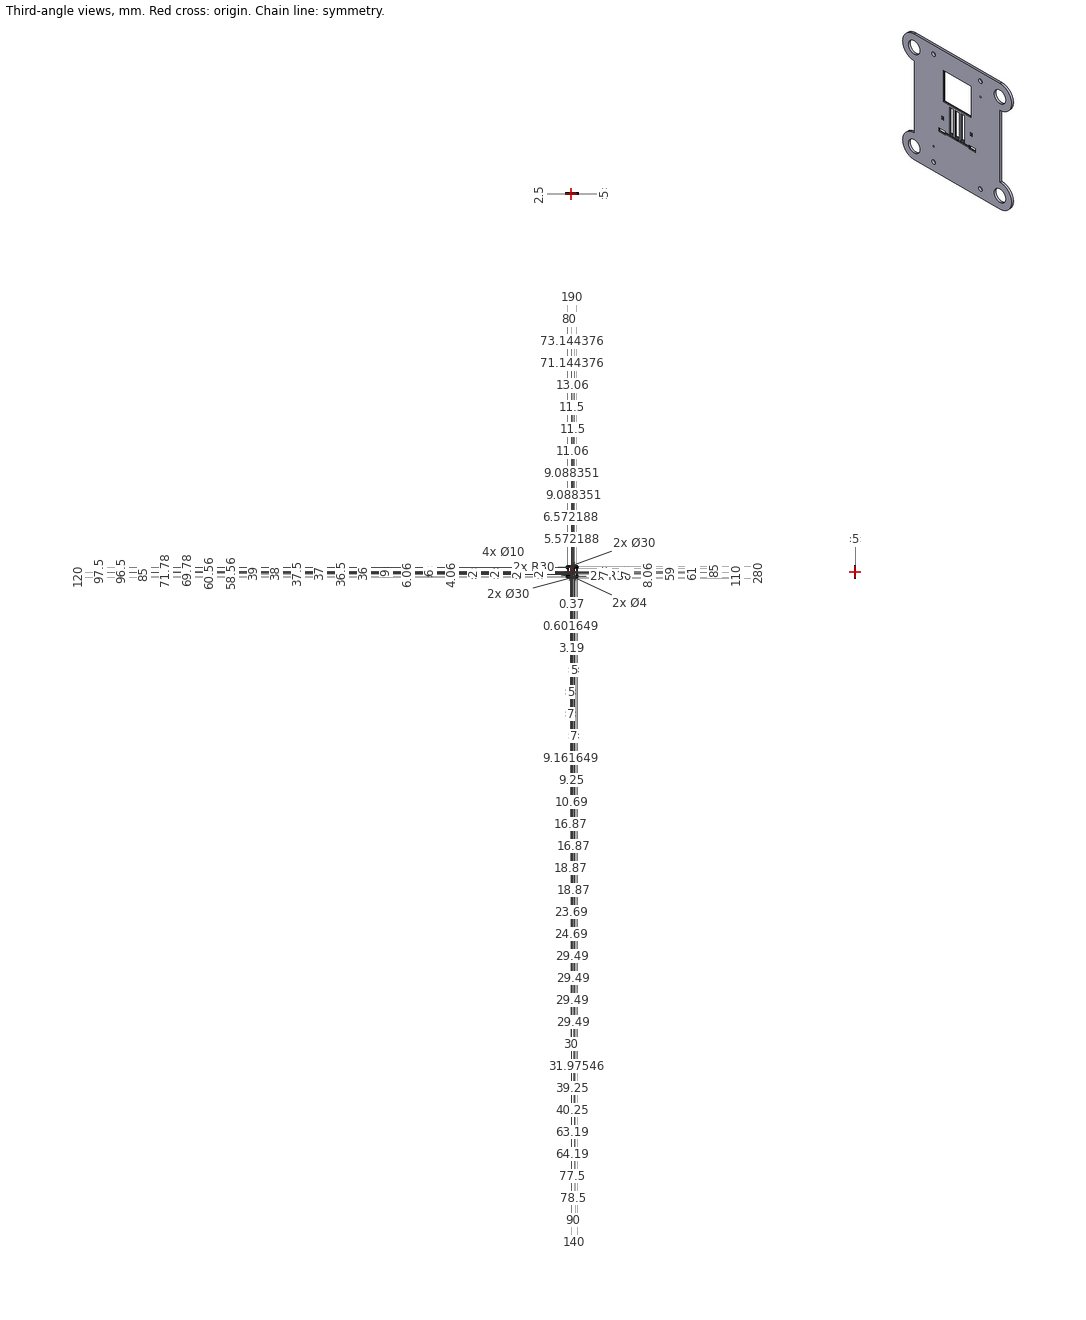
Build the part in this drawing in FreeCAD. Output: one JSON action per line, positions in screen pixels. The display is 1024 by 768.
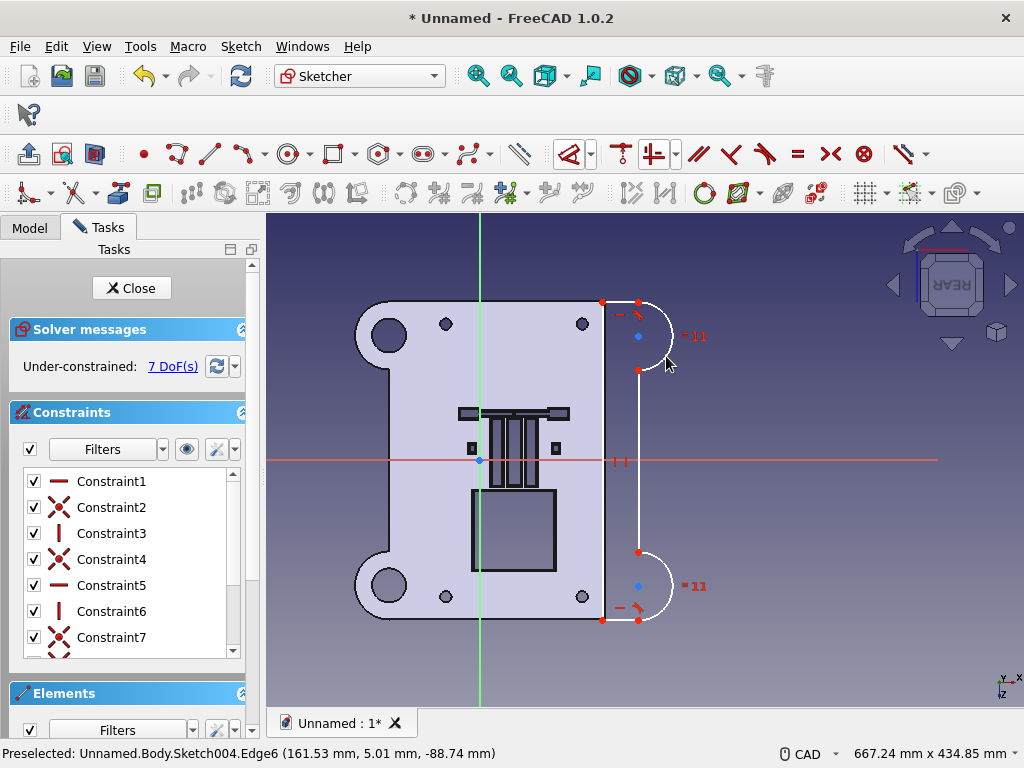
{"action": "left_click", "coordinate": [639, 586]}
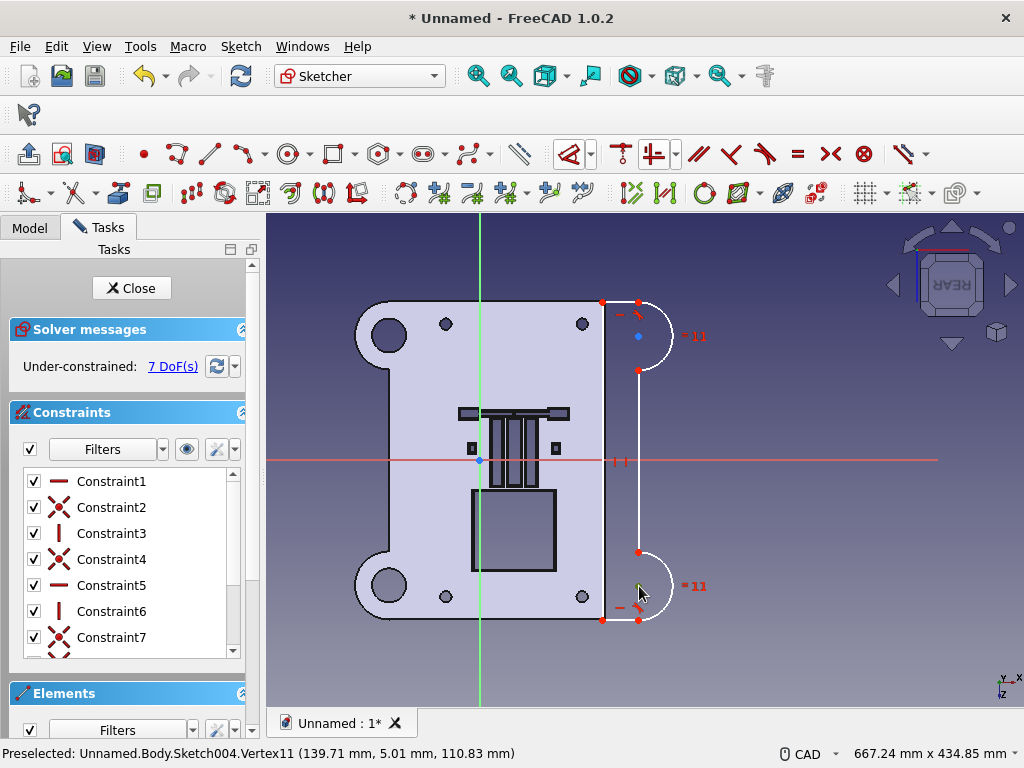
{"action": "left_click", "coordinate": [639, 336]}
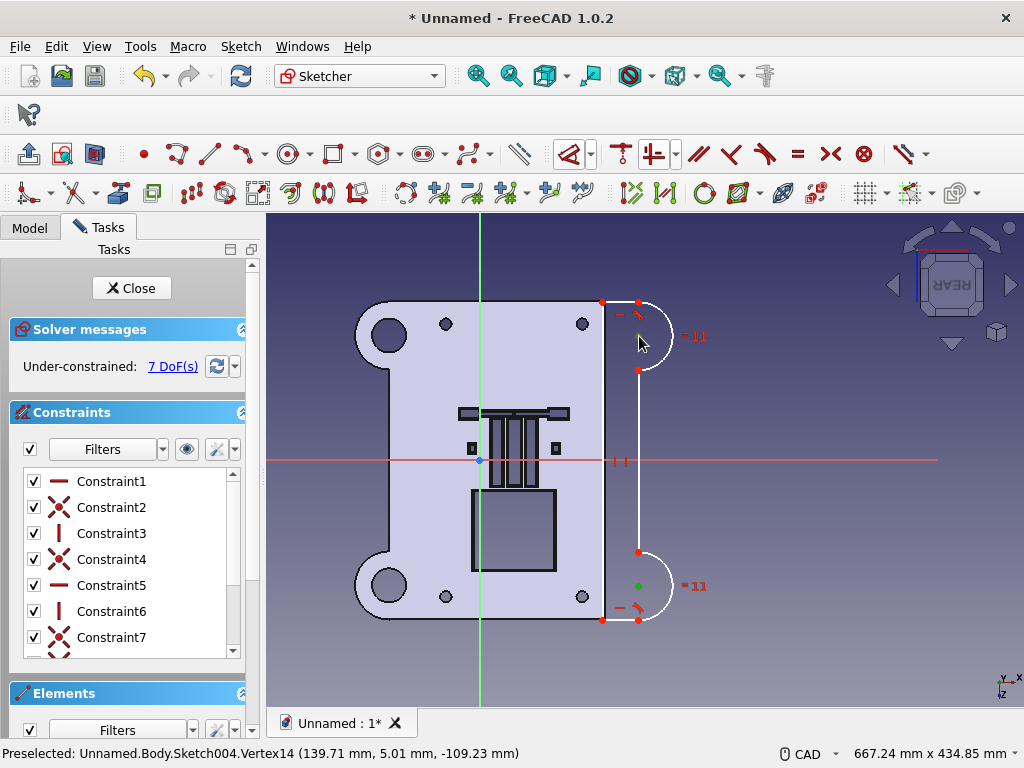
{"action": "left_click", "coordinate": [334, 460]}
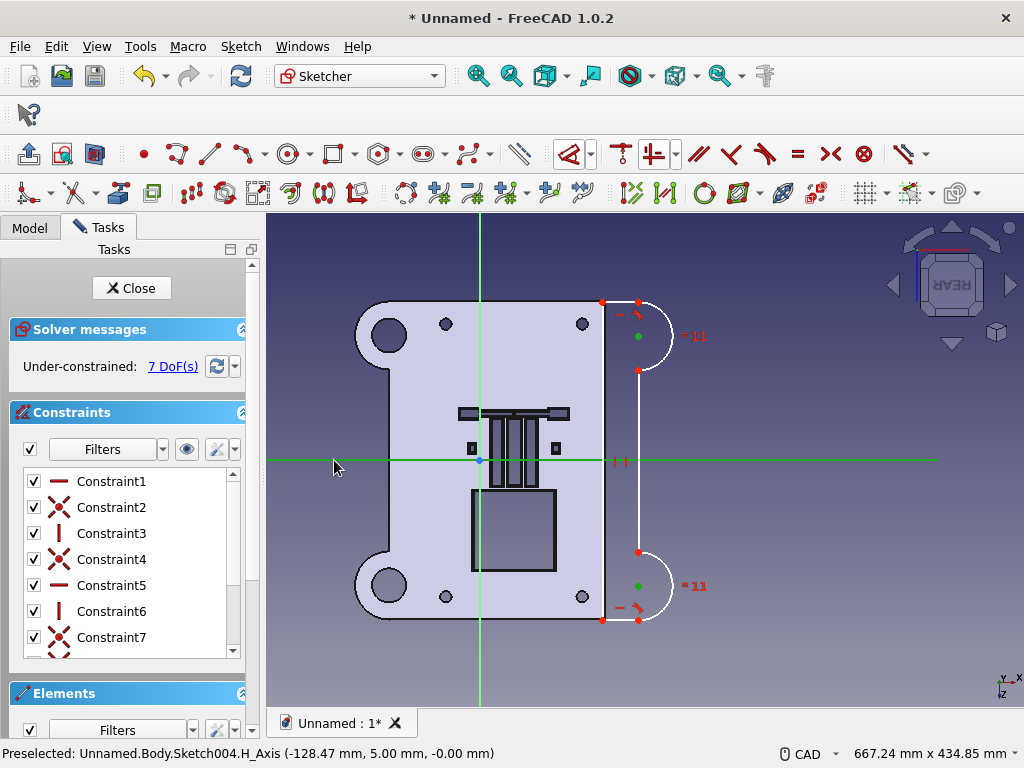
{"action": "left_click", "coordinate": [831, 154]}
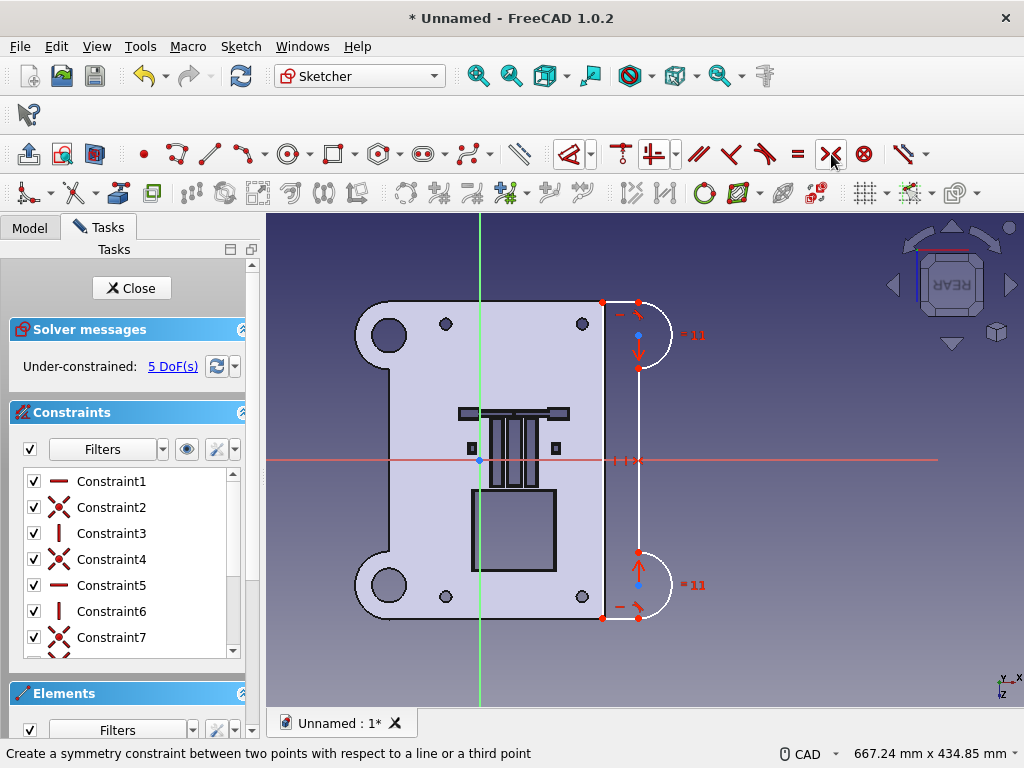
{"action": "left_click", "coordinate": [665, 605]}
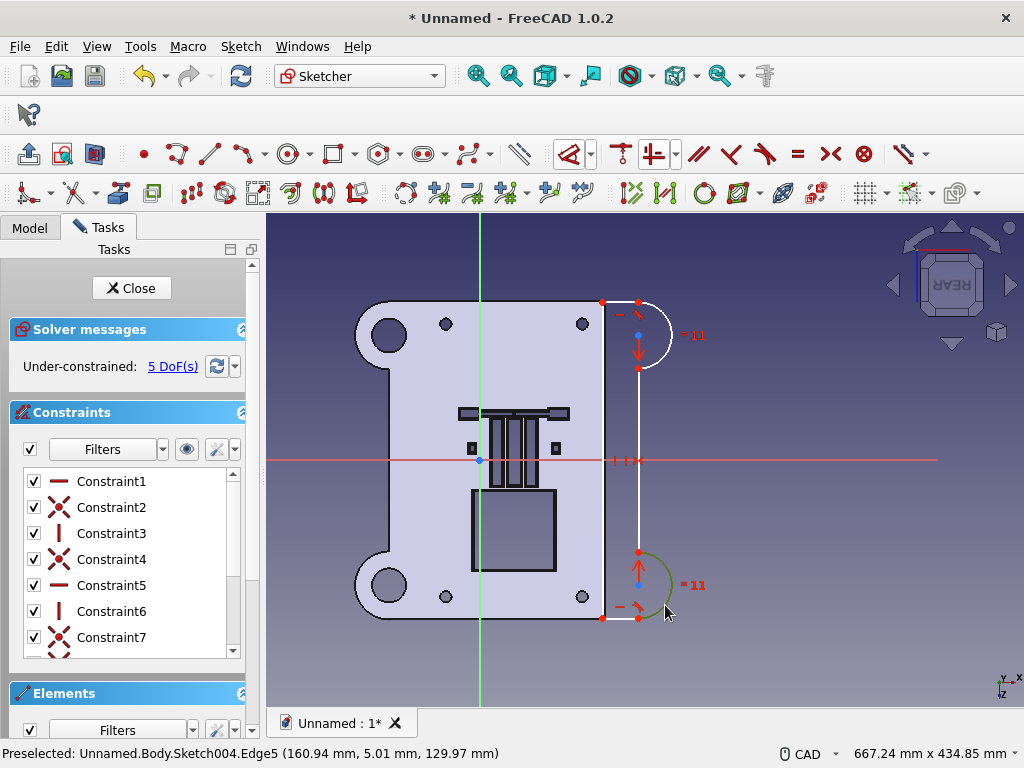
{"action": "left_click", "coordinate": [590, 154]}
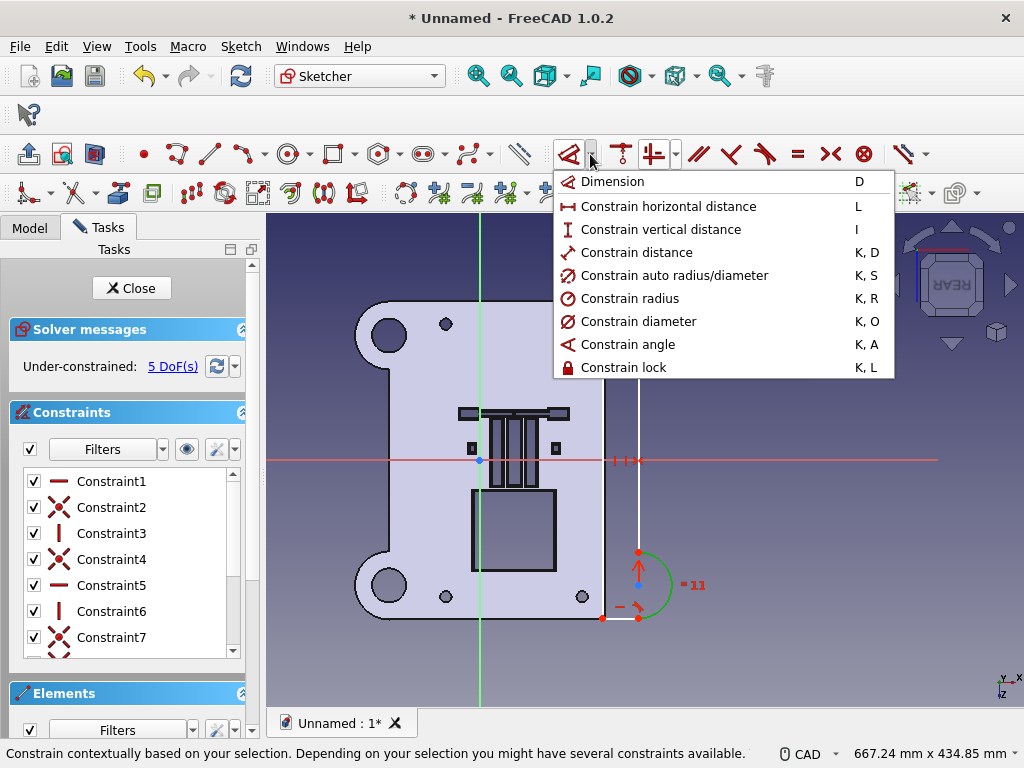
{"action": "left_click", "coordinate": [724, 298]}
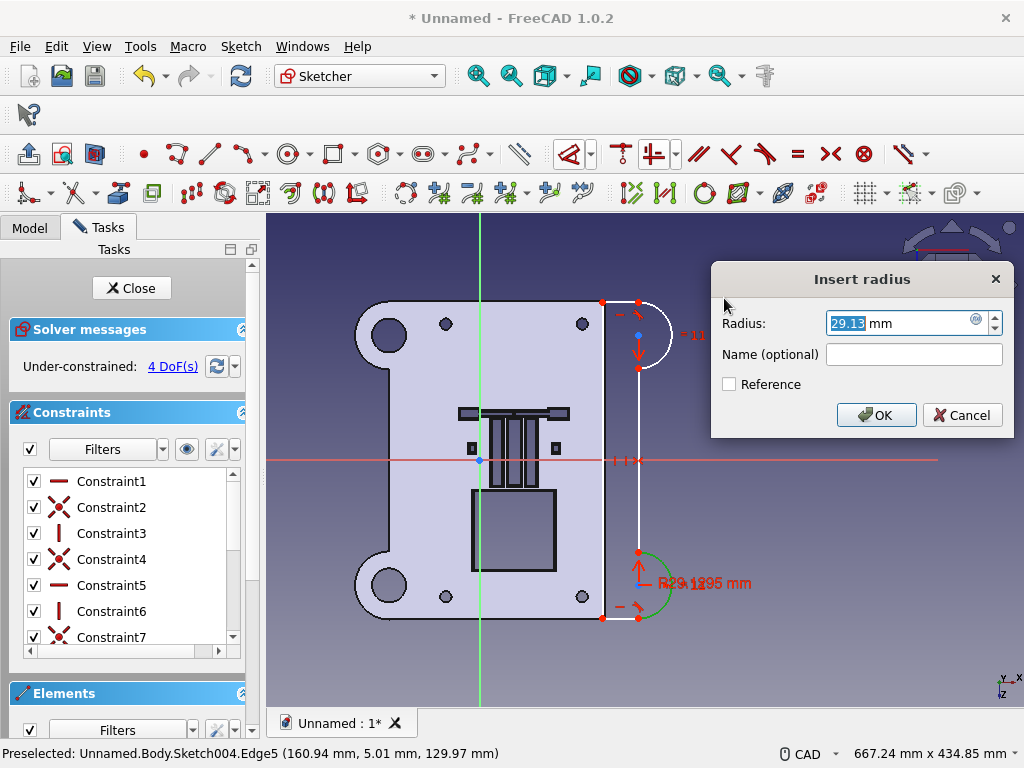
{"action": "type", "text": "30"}
{"action": "key", "text": "Return"}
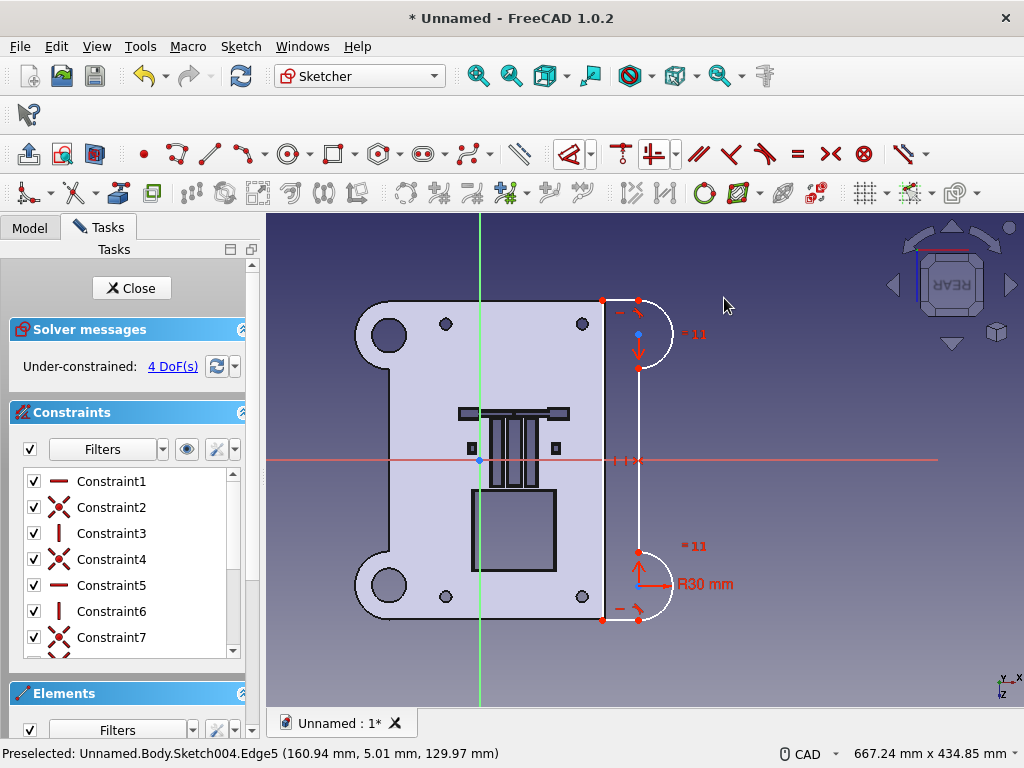
{"action": "left_click", "coordinate": [603, 396]}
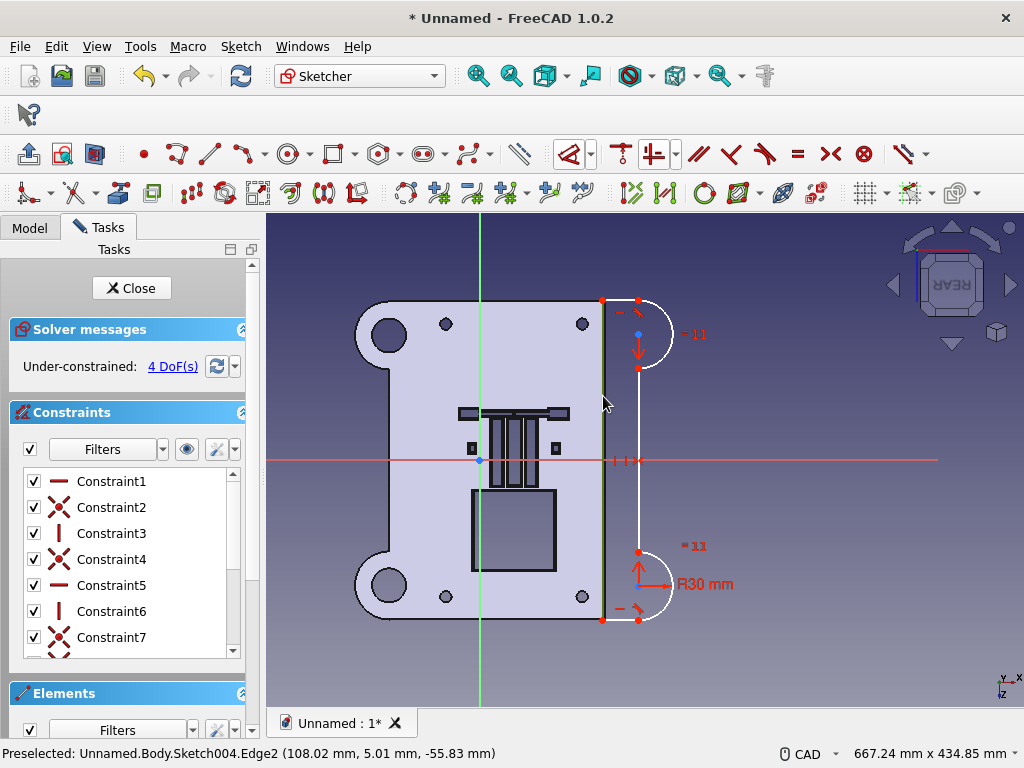
{"action": "left_click", "coordinate": [590, 154]}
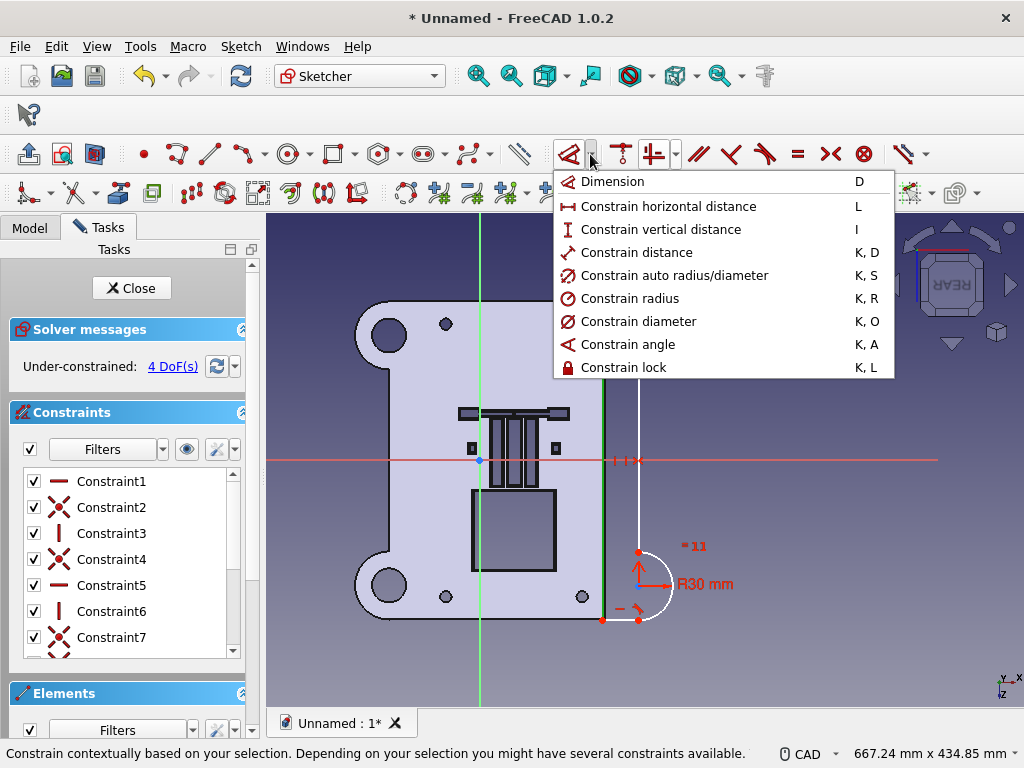
{"action": "left_click", "coordinate": [724, 230]}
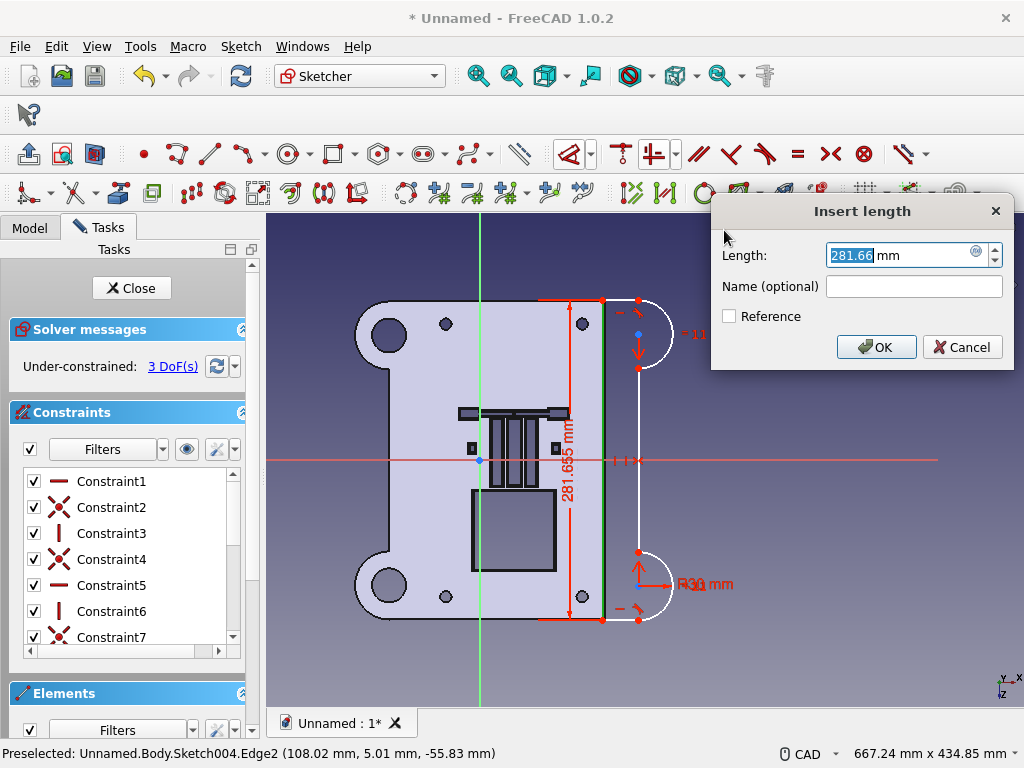
{"action": "type", "text": "280"}
{"action": "key", "text": "Return"}